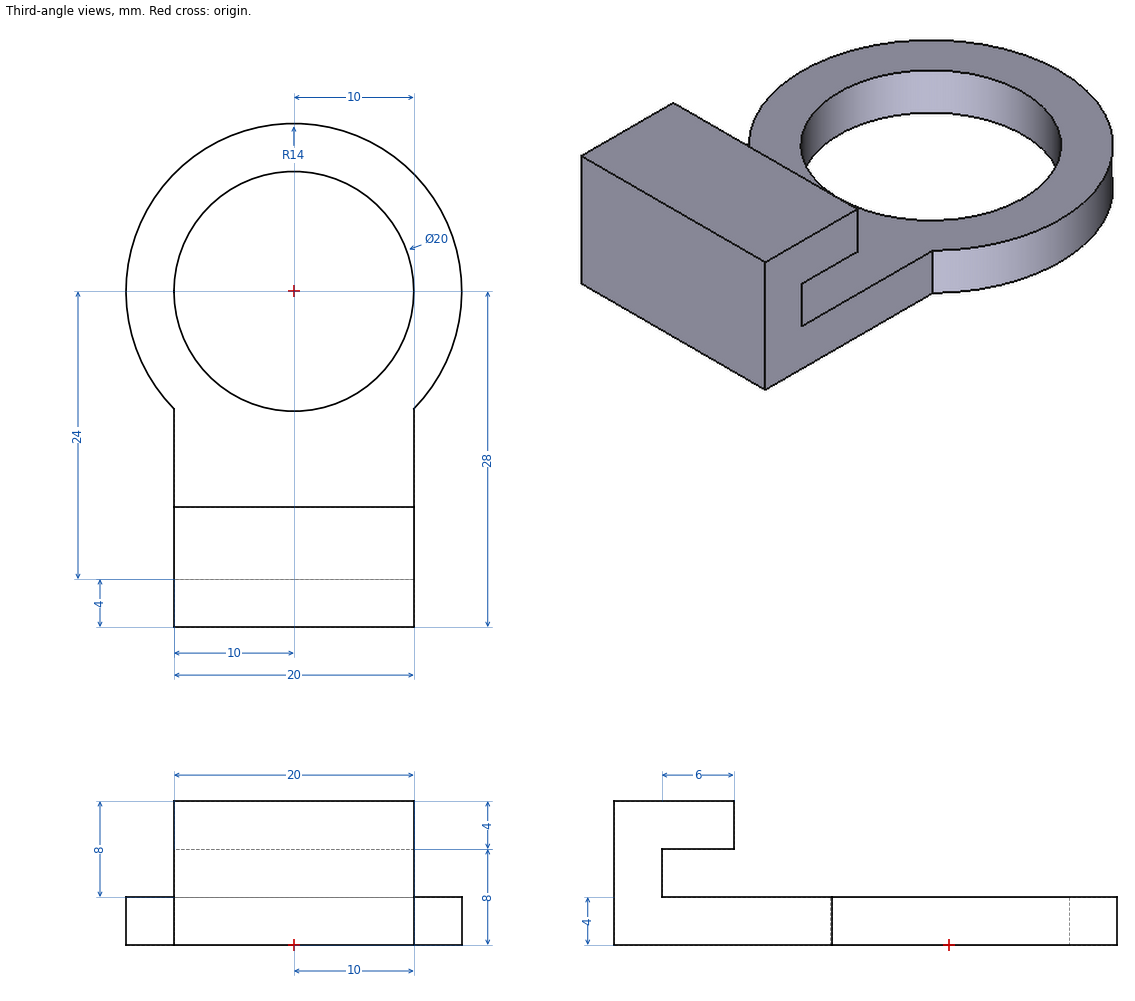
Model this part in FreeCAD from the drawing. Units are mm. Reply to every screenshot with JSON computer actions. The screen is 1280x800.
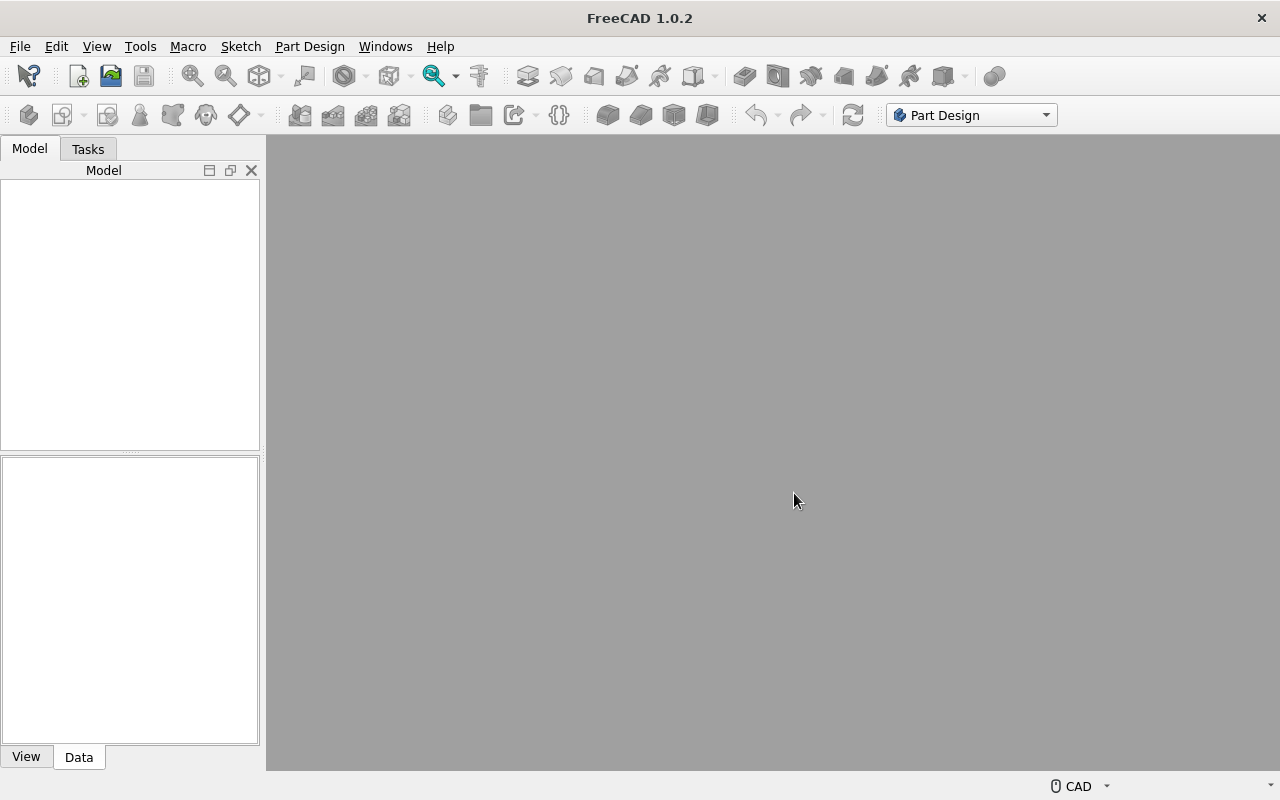
{"action": "left_click", "coordinate": [78, 76]}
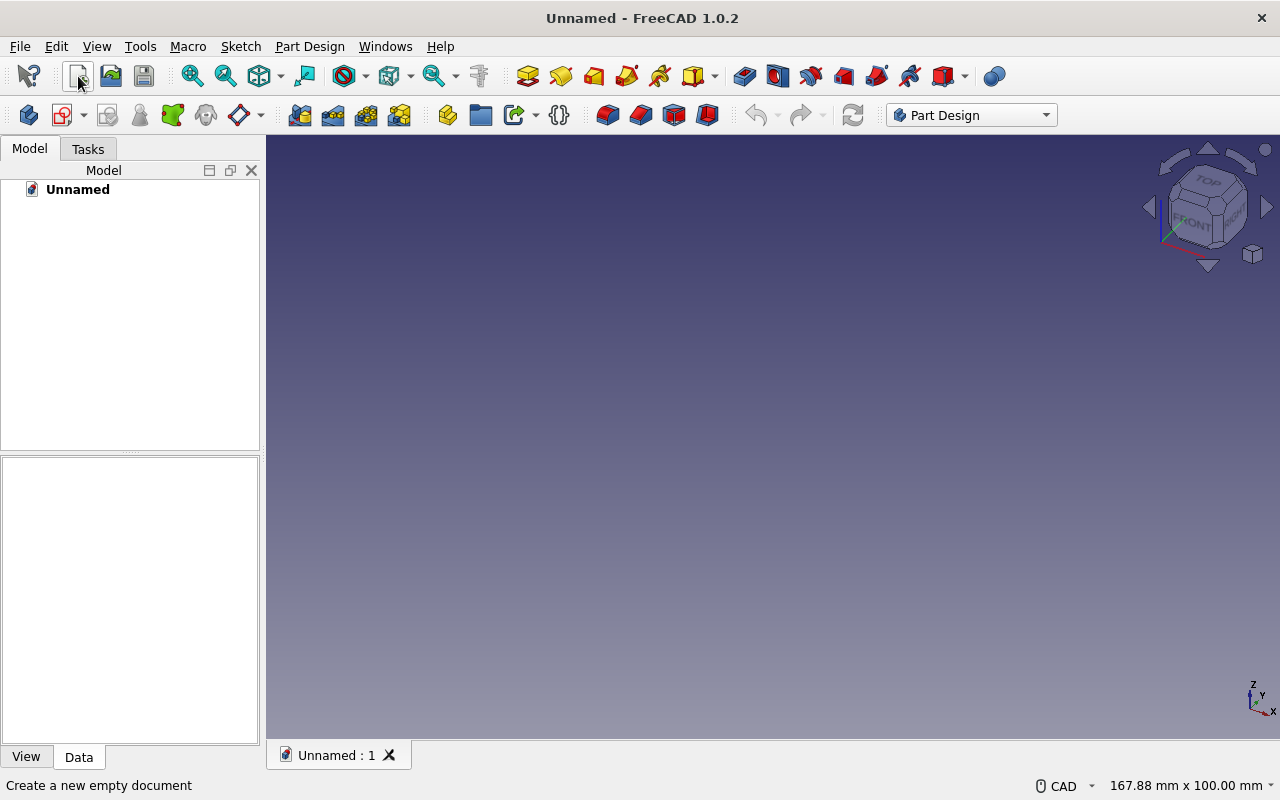
{"action": "left_click", "coordinate": [62, 116]}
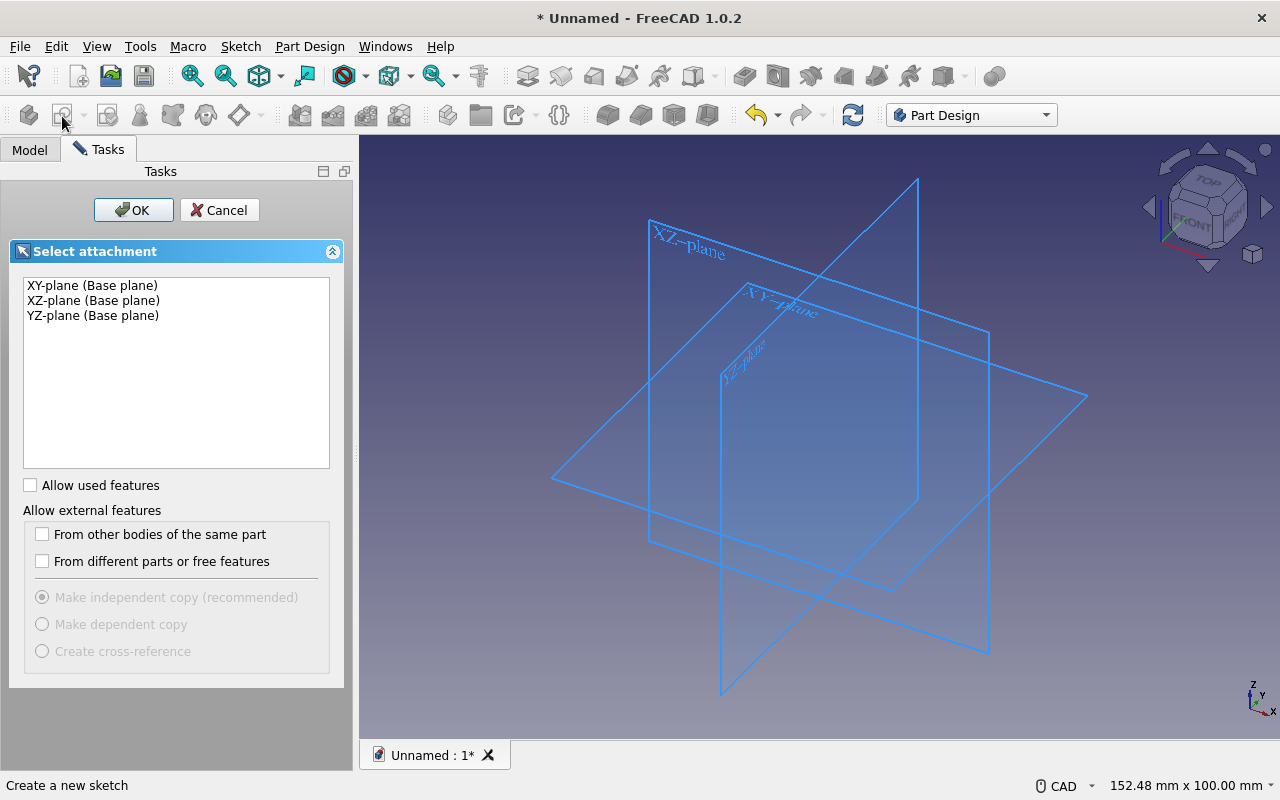
{"action": "left_click", "coordinate": [84, 286]}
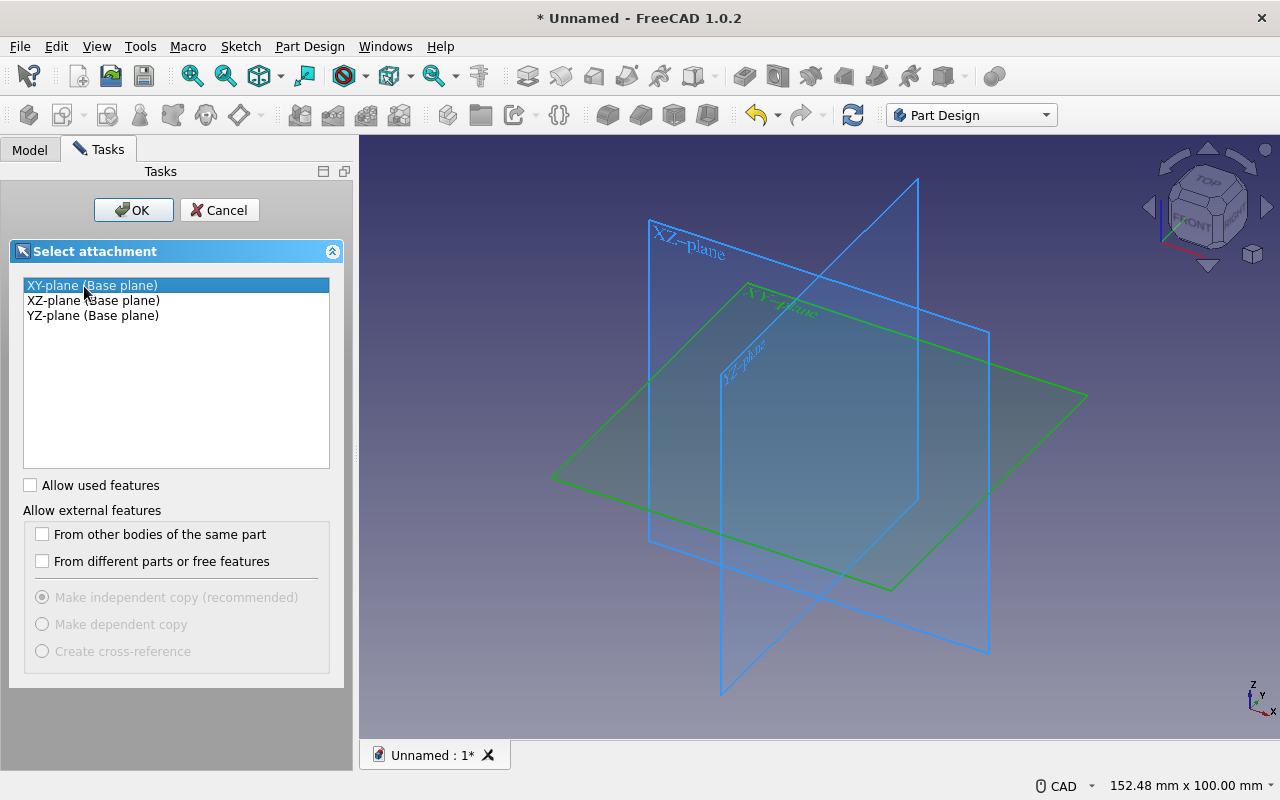
{"action": "left_click", "coordinate": [134, 210]}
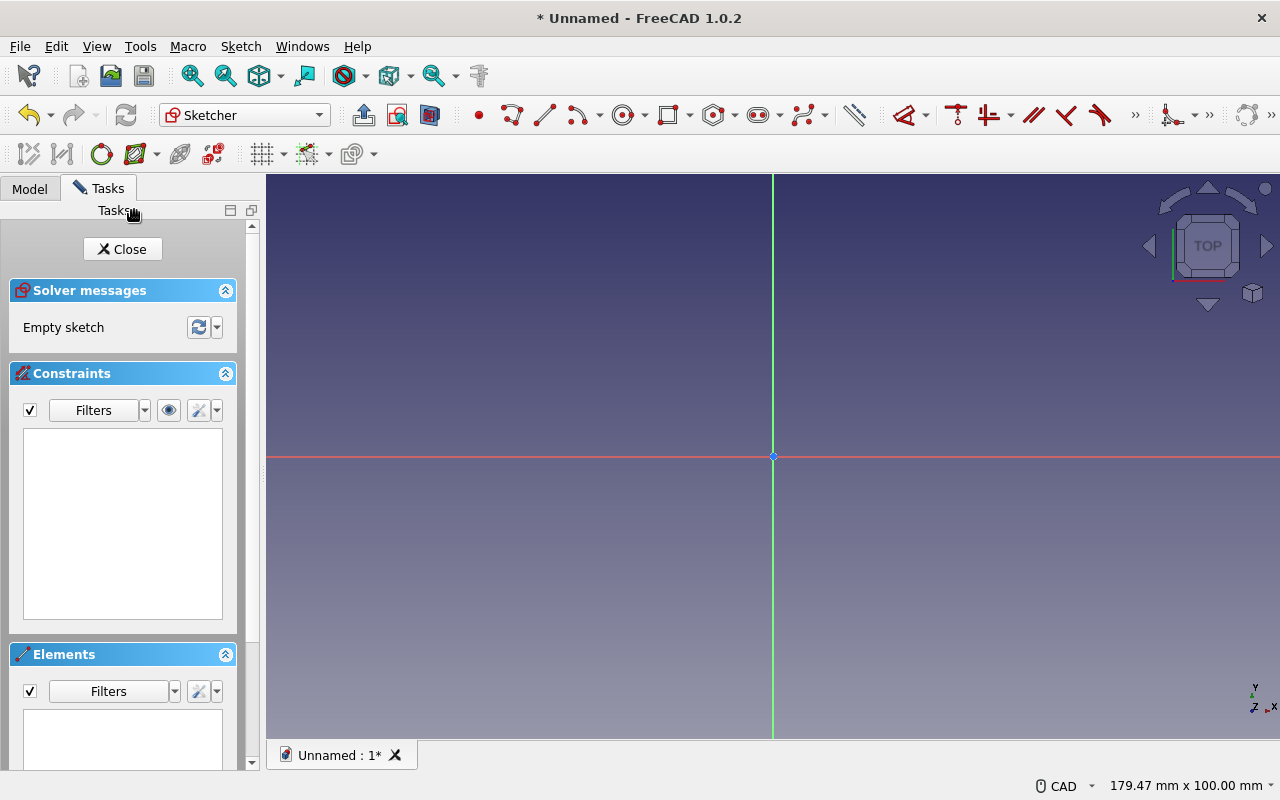
{"action": "scroll", "coordinate": [912, 576], "scroll_direction": "up", "scroll_amount": 2}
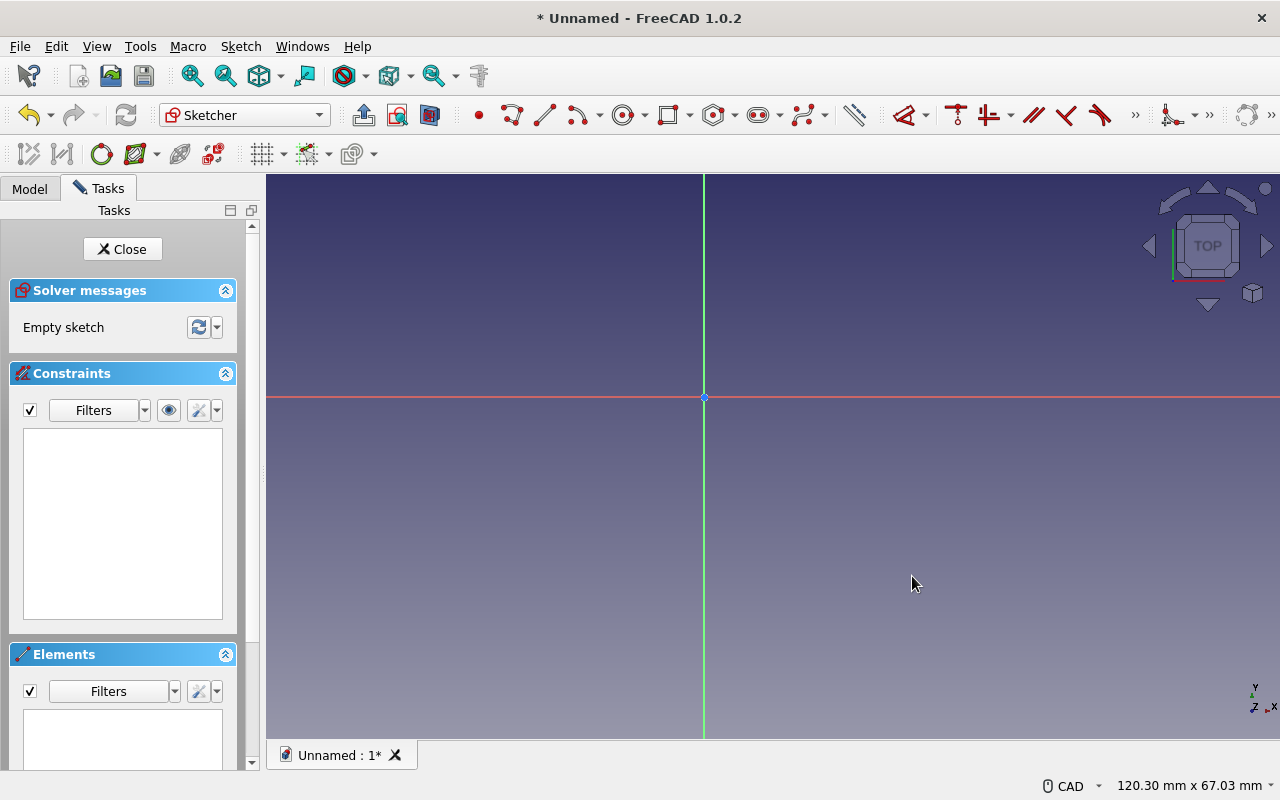
{"action": "key", "text": "g m"}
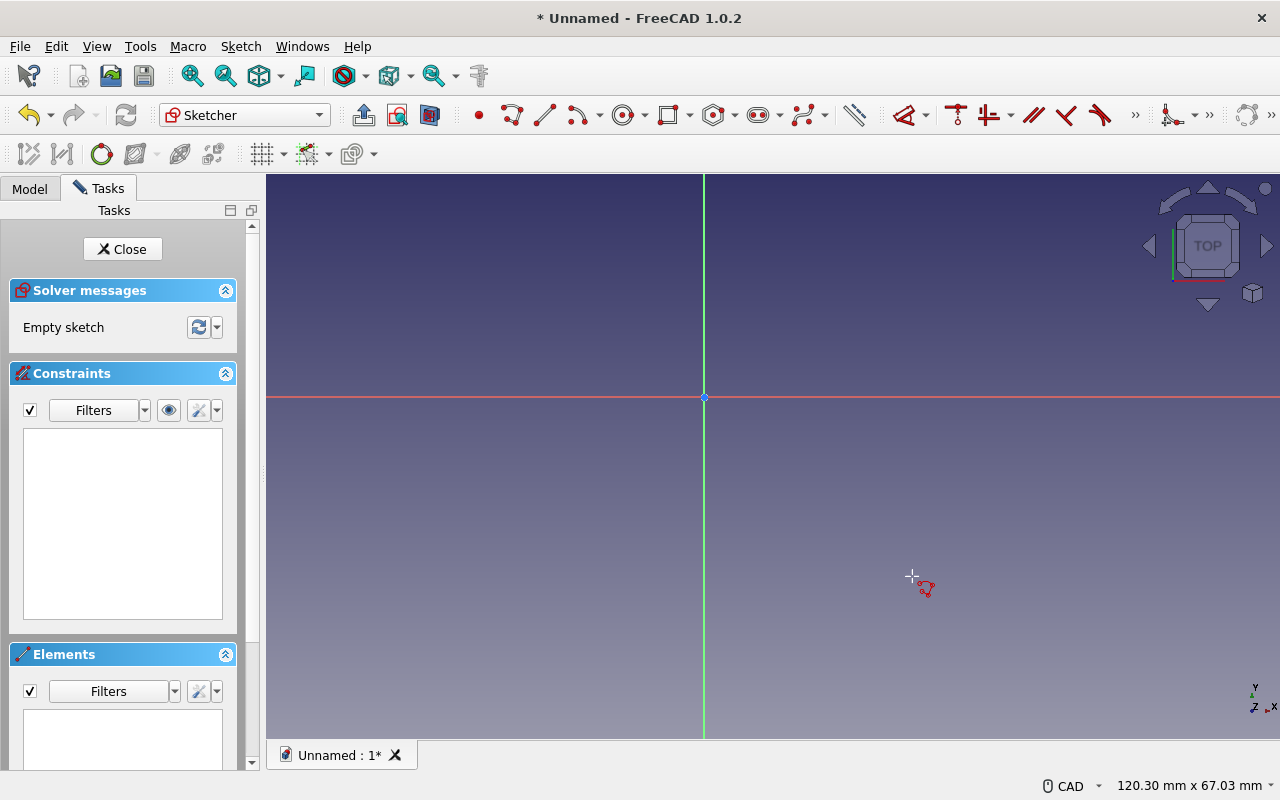
{"action": "left_click", "coordinate": [789, 480]}
{"action": "left_click", "coordinate": [789, 633]}
{"action": "left_click", "coordinate": [620, 633]}
{"action": "left_click", "coordinate": [620, 480]}
{"action": "right_click", "coordinate": [620, 480]}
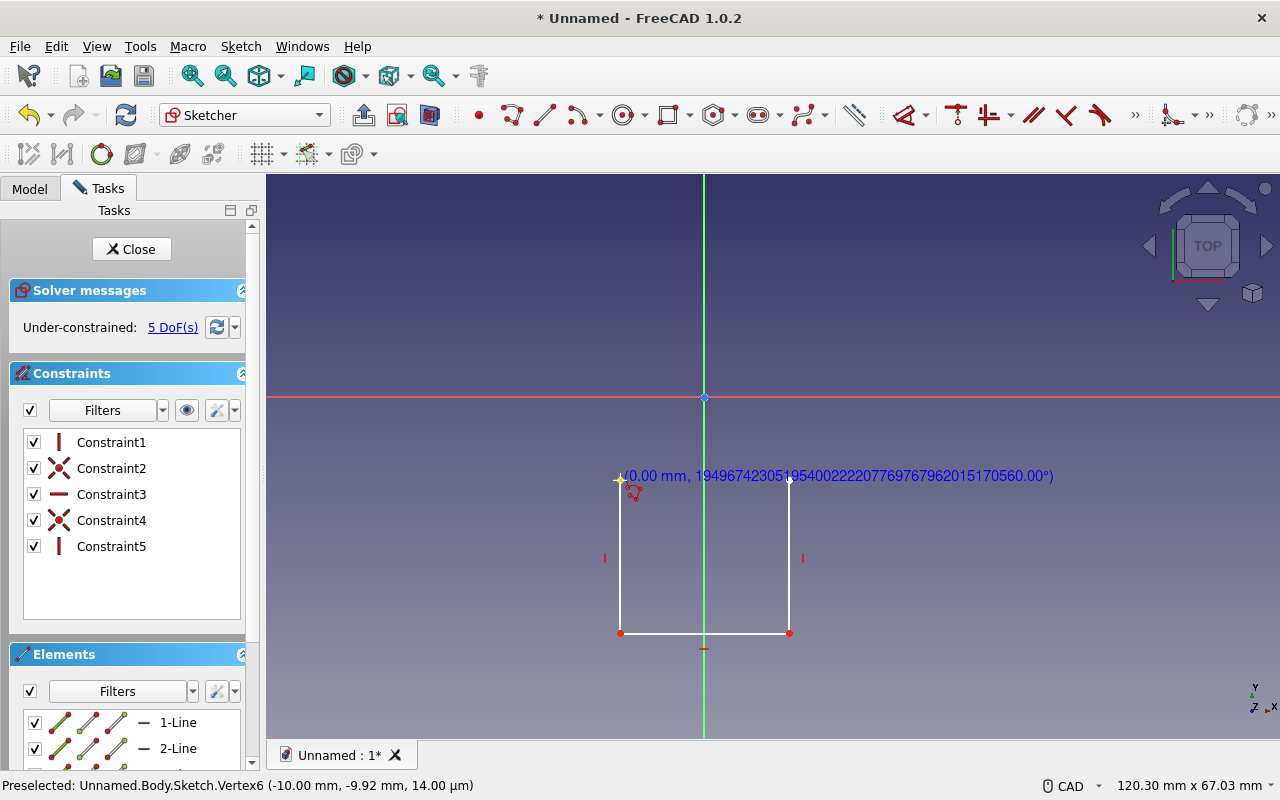
{"action": "key", "text": "g 3 a"}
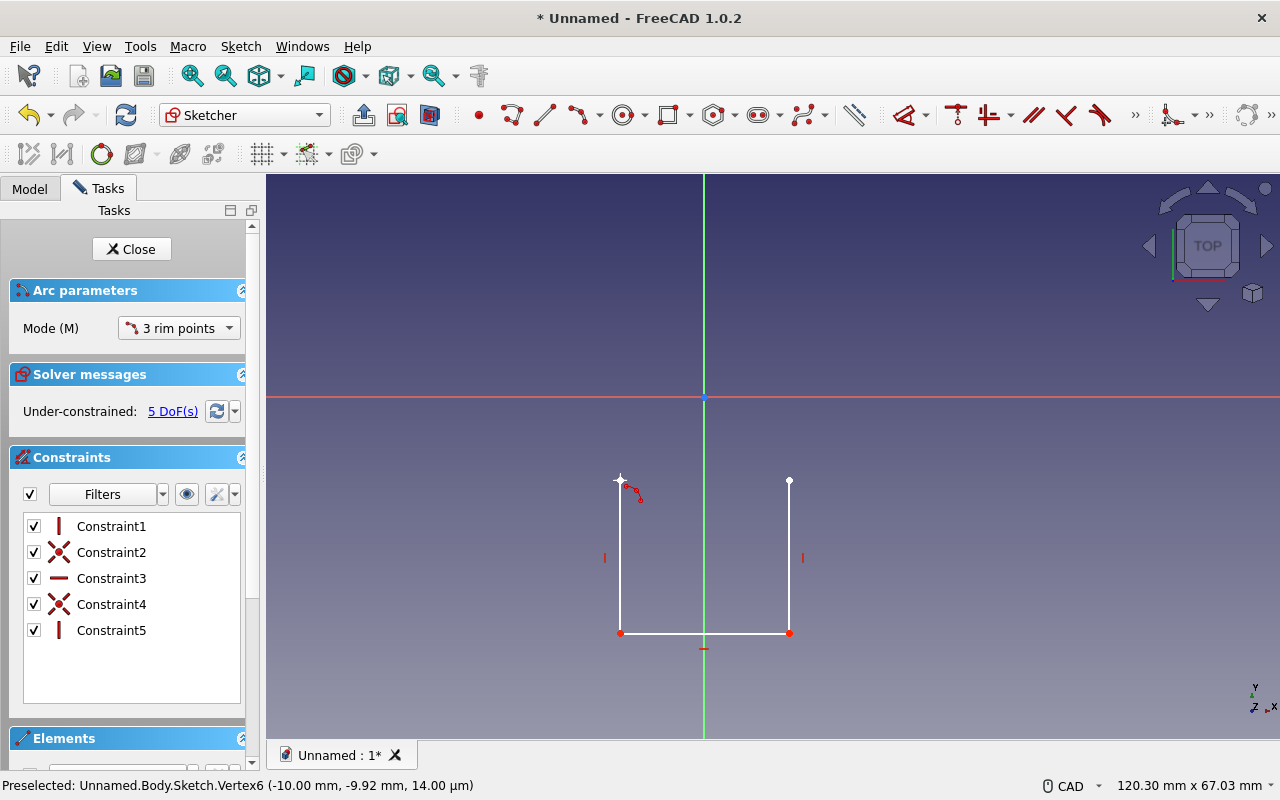
{"action": "left_click", "coordinate": [620, 481]}
{"action": "left_click", "coordinate": [789, 481]}
{"action": "left_click", "coordinate": [758, 292]}
{"action": "key", "text": "Escape"}